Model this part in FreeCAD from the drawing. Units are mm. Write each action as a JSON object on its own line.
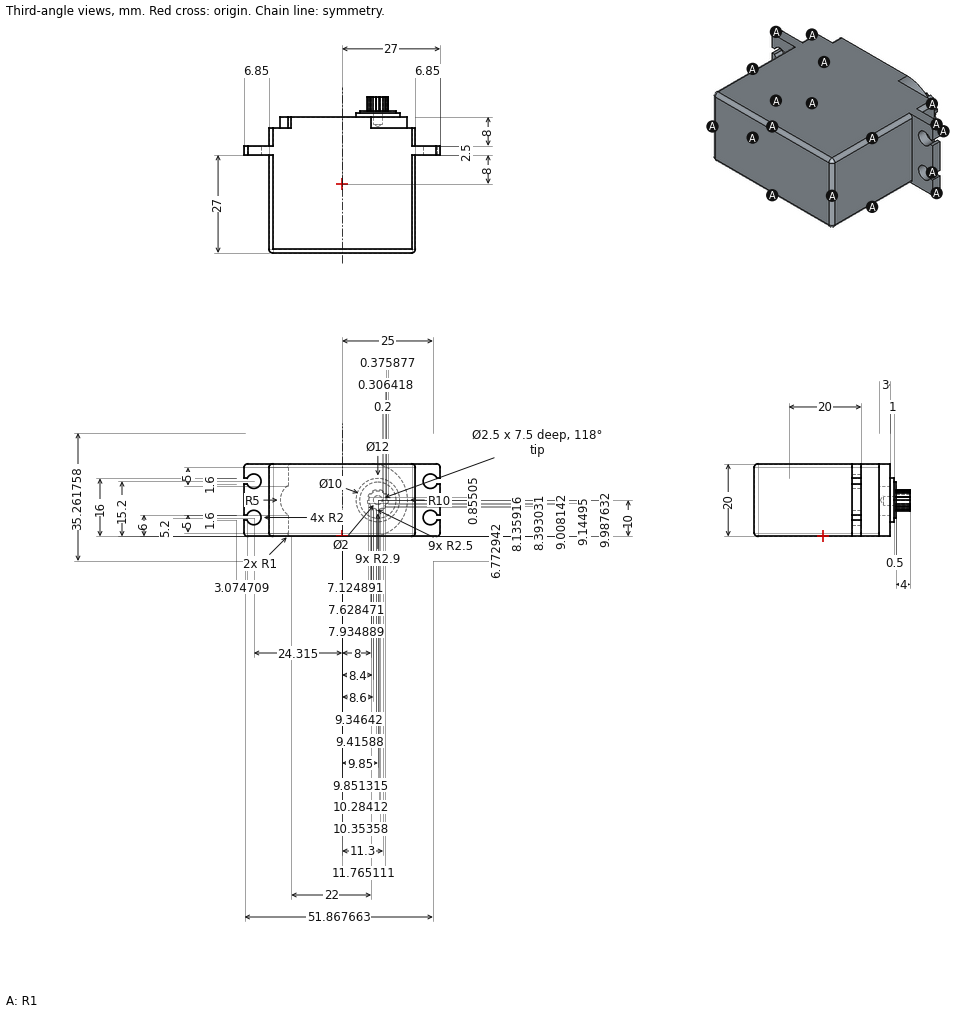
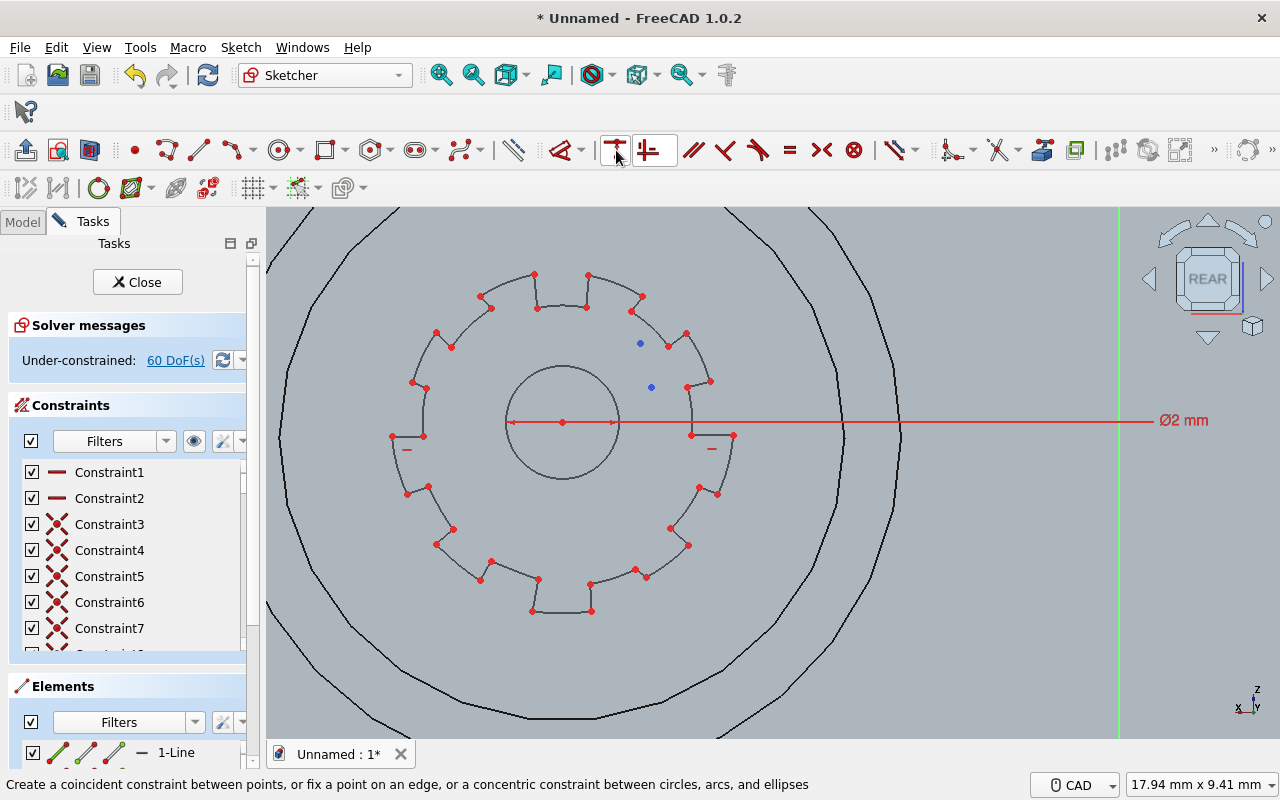
{"action": "left_click", "coordinate": [602, 382]}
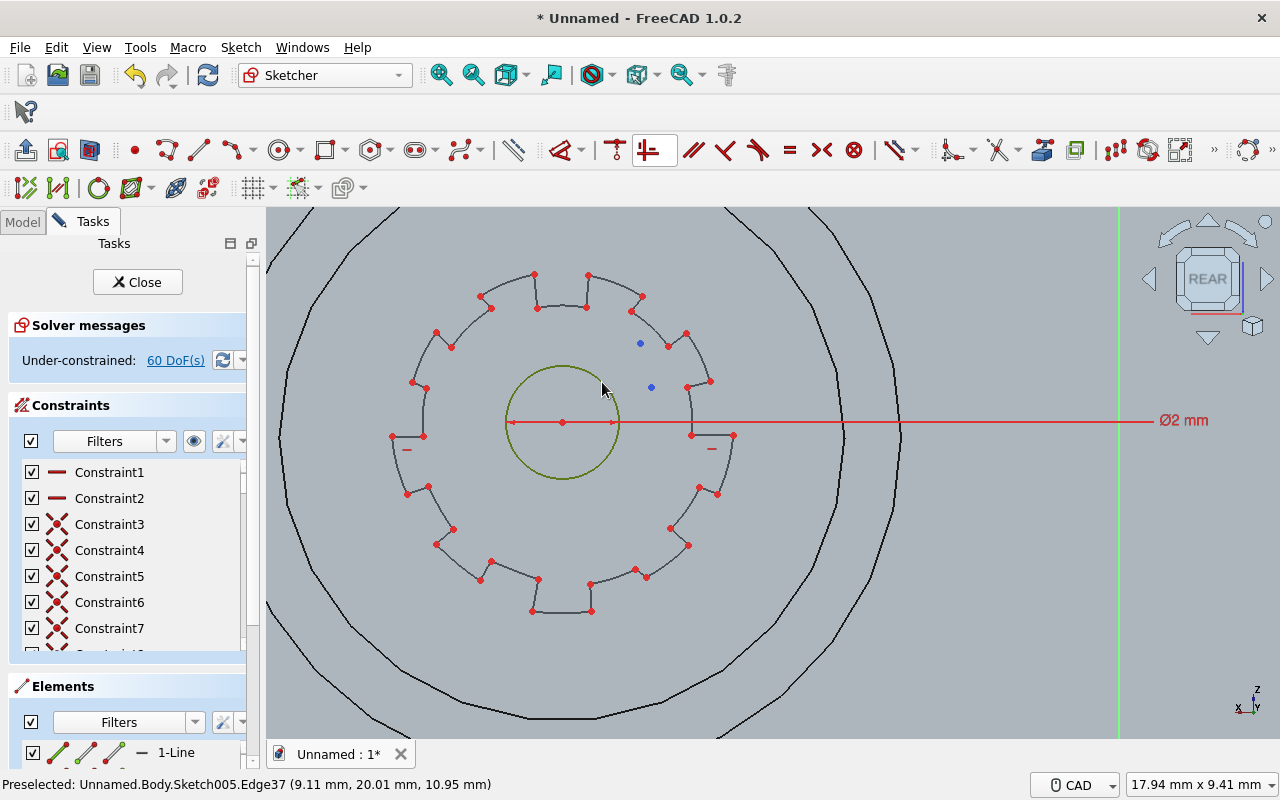
{"action": "left_click", "coordinate": [435, 500]}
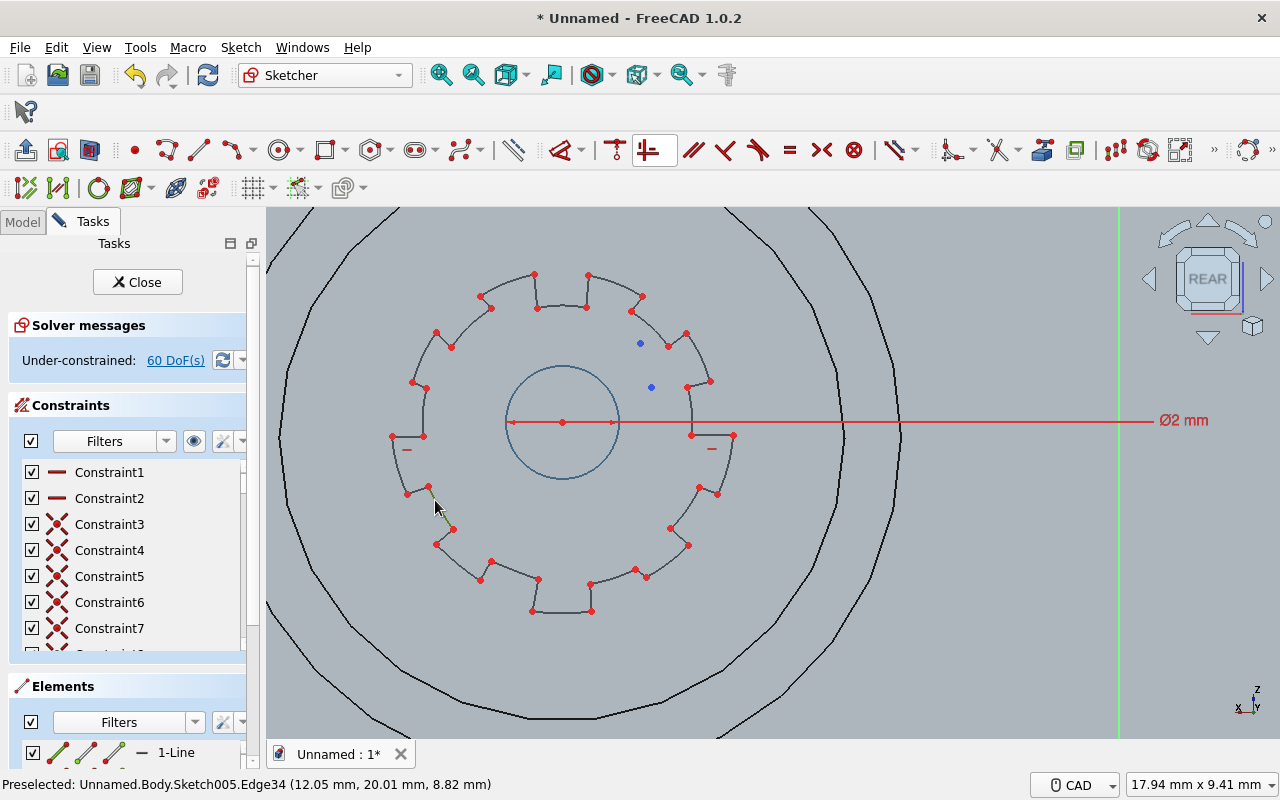
{"action": "key", "text": "c"}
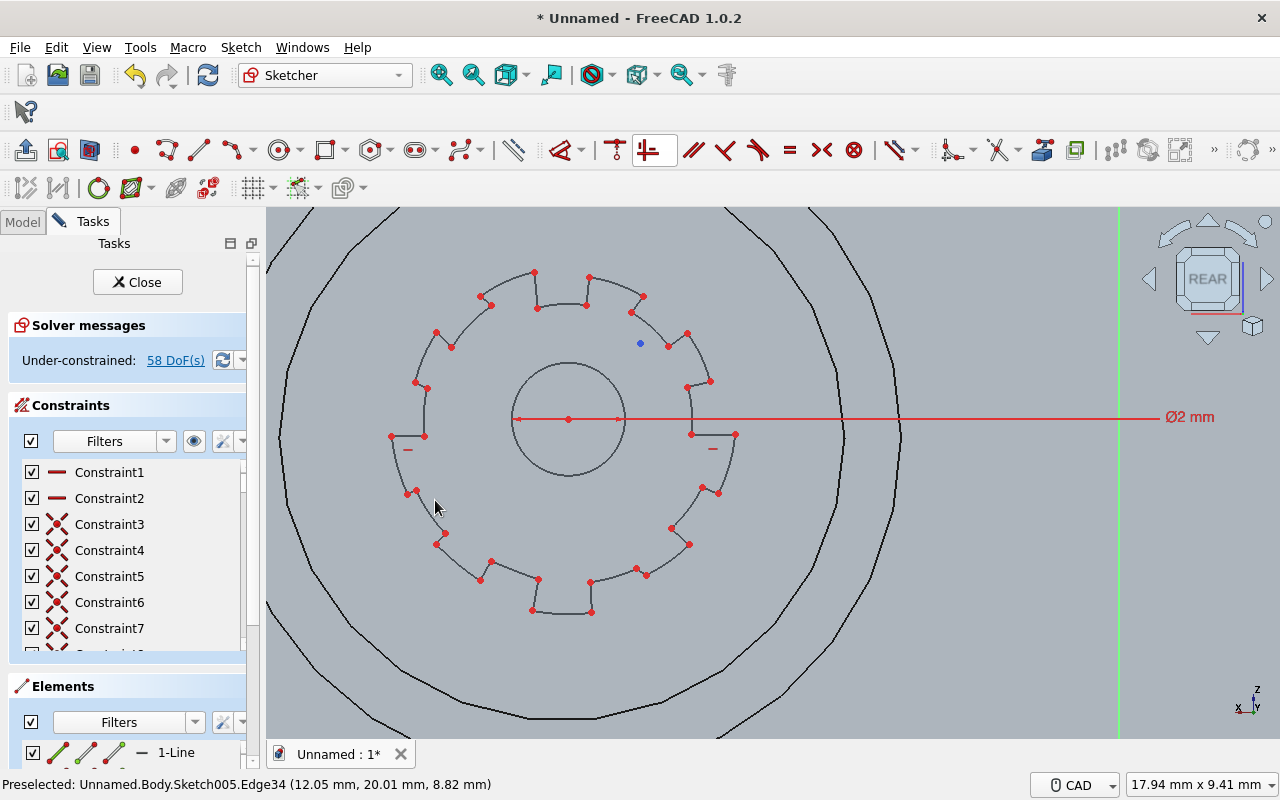
{"action": "left_click", "coordinate": [608, 379]}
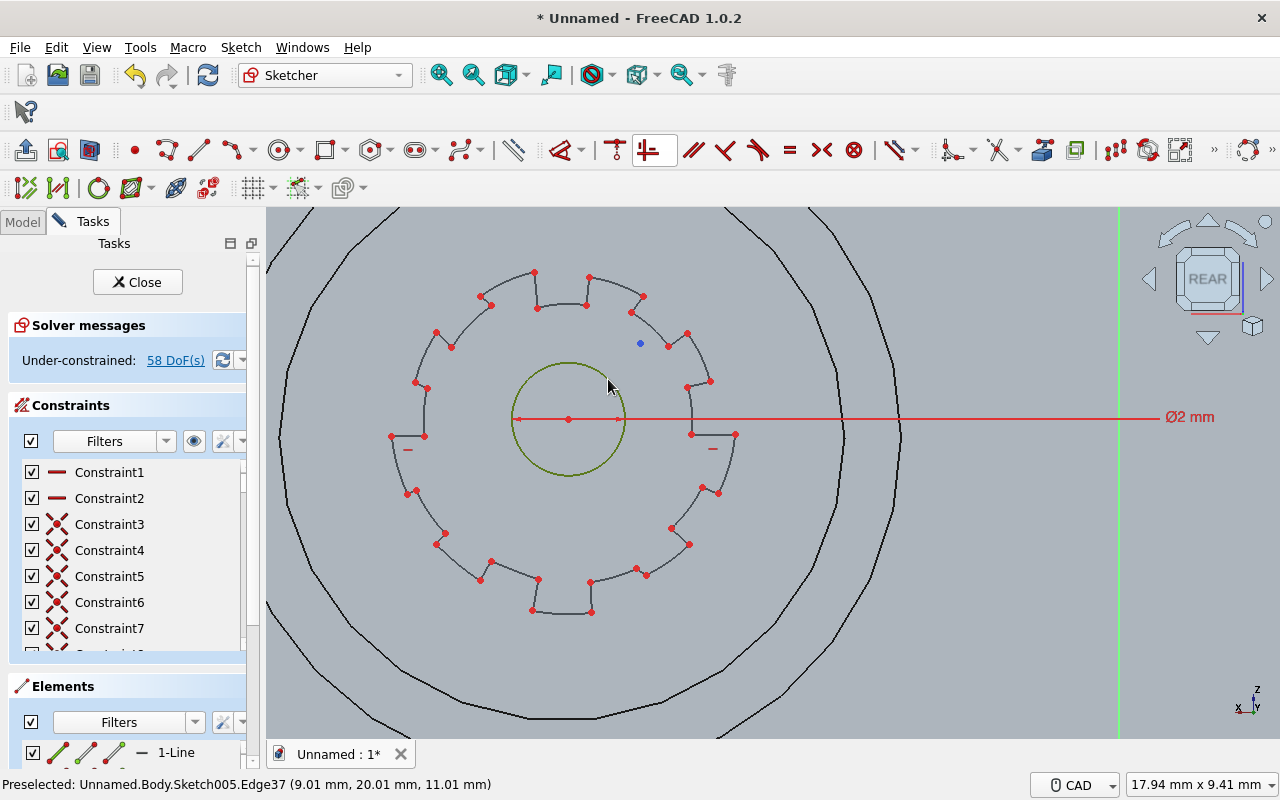
{"action": "left_click", "coordinate": [448, 556]}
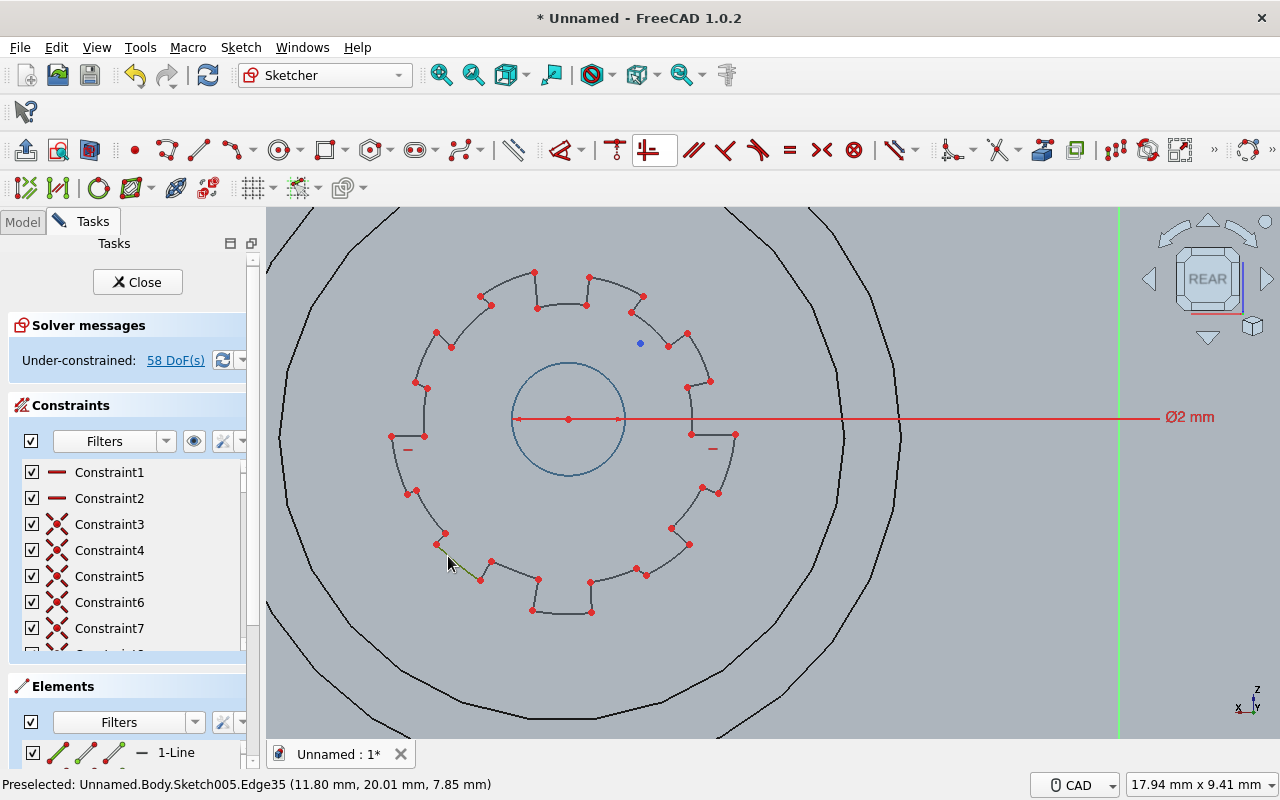
{"action": "left_click", "coordinate": [616, 150]}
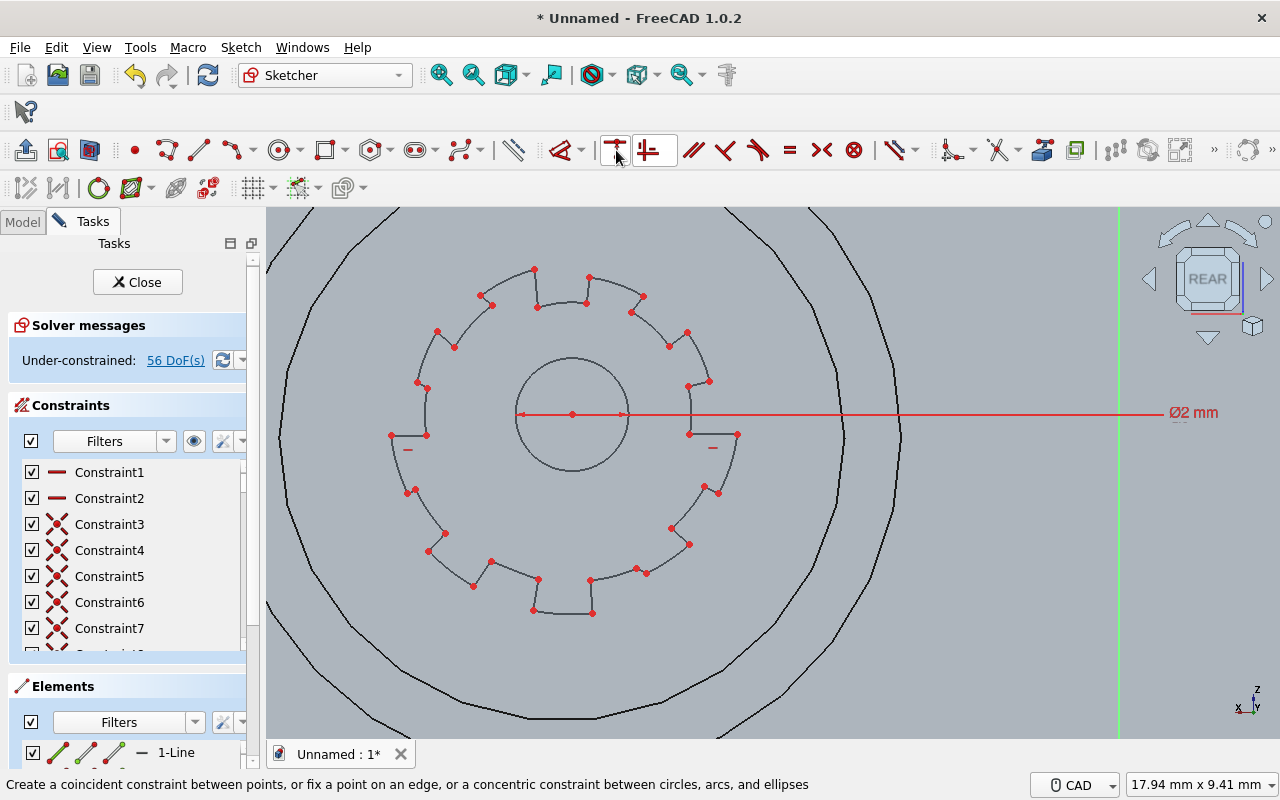
{"action": "left_click", "coordinate": [612, 375]}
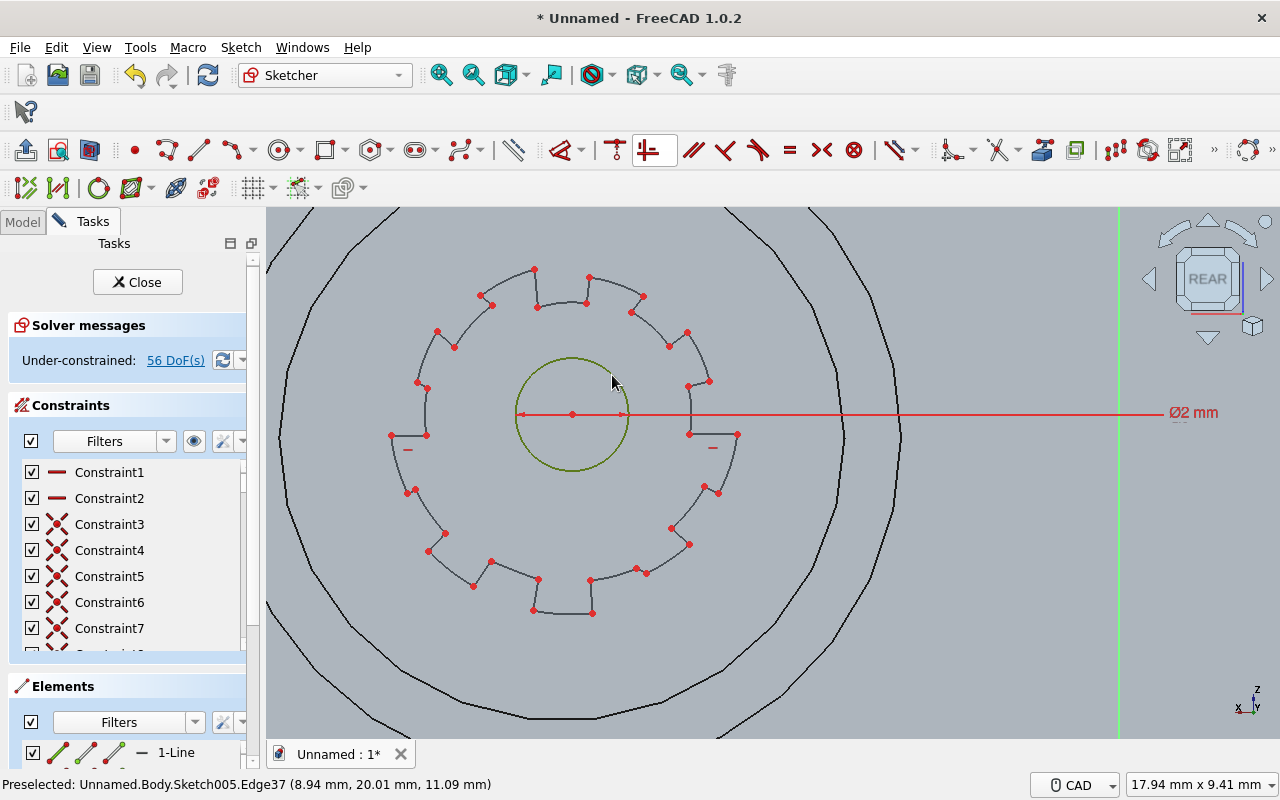
{"action": "left_click", "coordinate": [505, 567]}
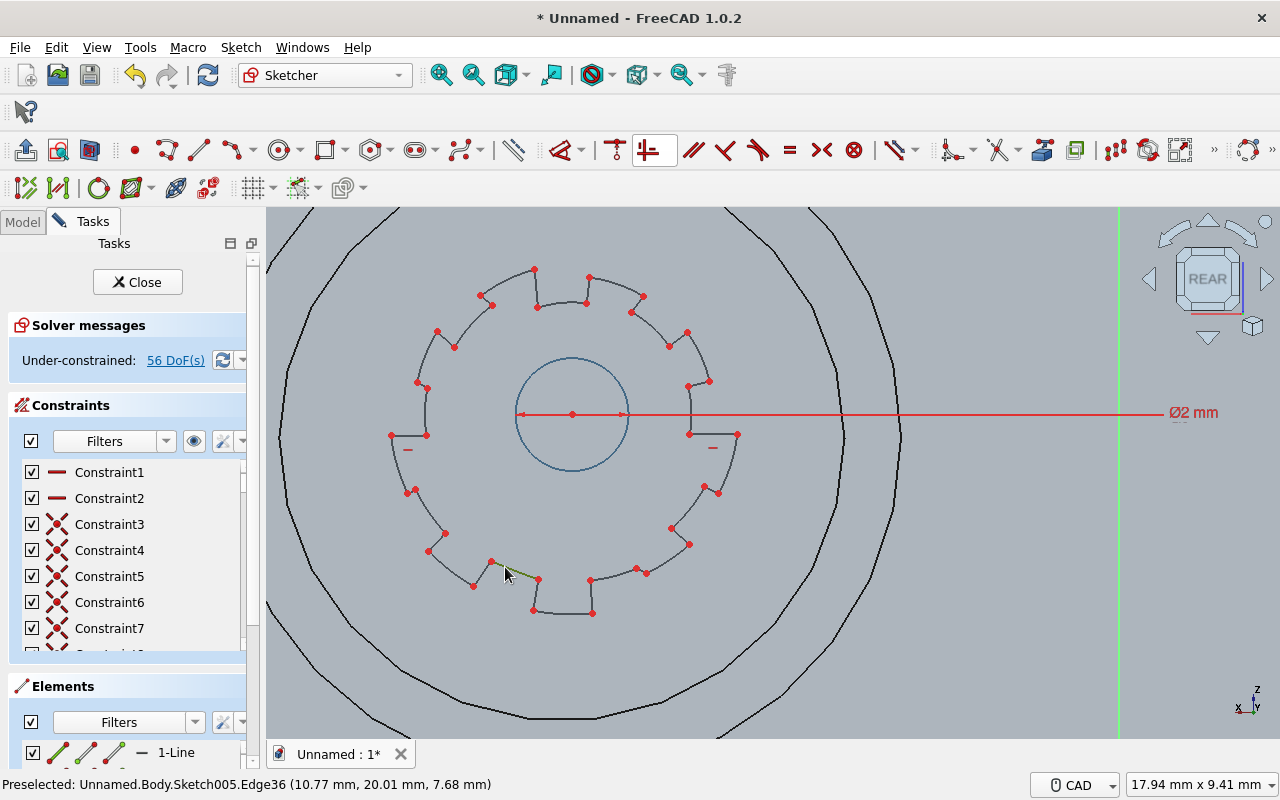
{"action": "key", "text": "c"}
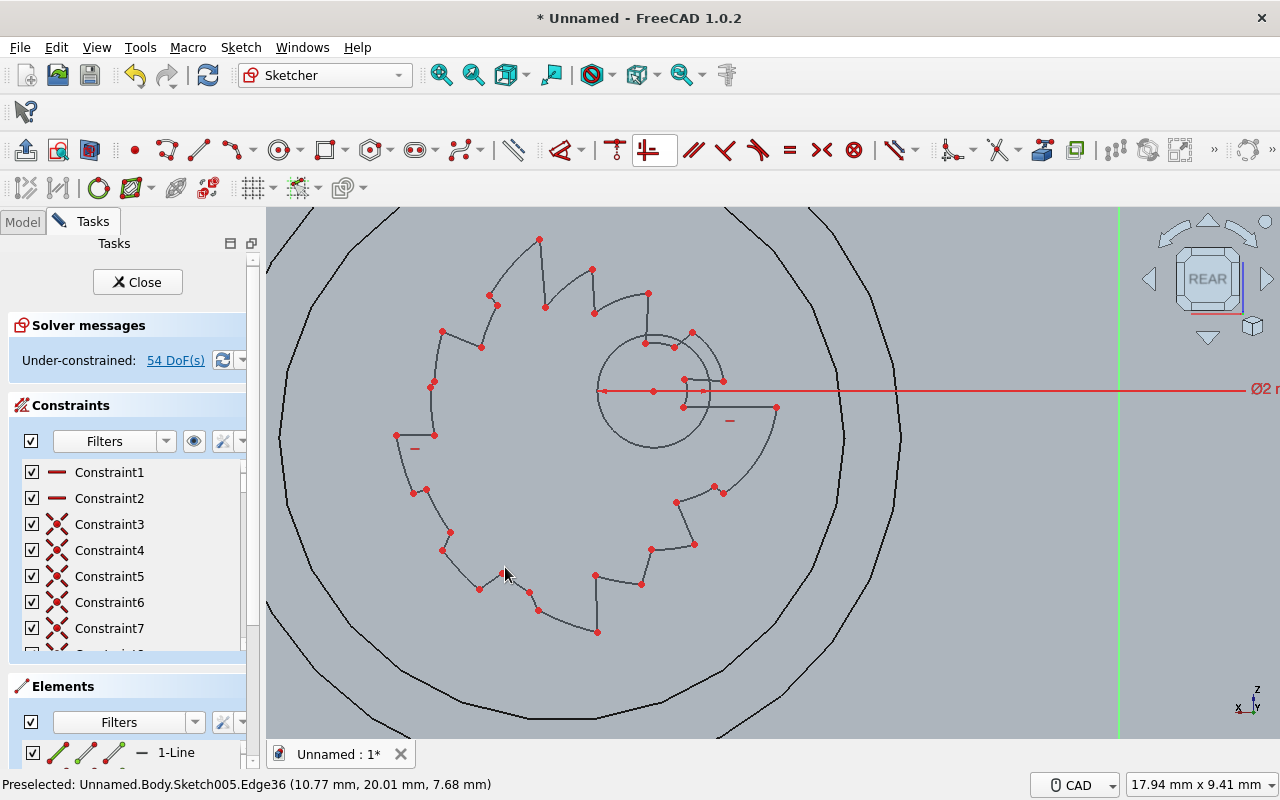
{"action": "left_click", "coordinate": [555, 618]}